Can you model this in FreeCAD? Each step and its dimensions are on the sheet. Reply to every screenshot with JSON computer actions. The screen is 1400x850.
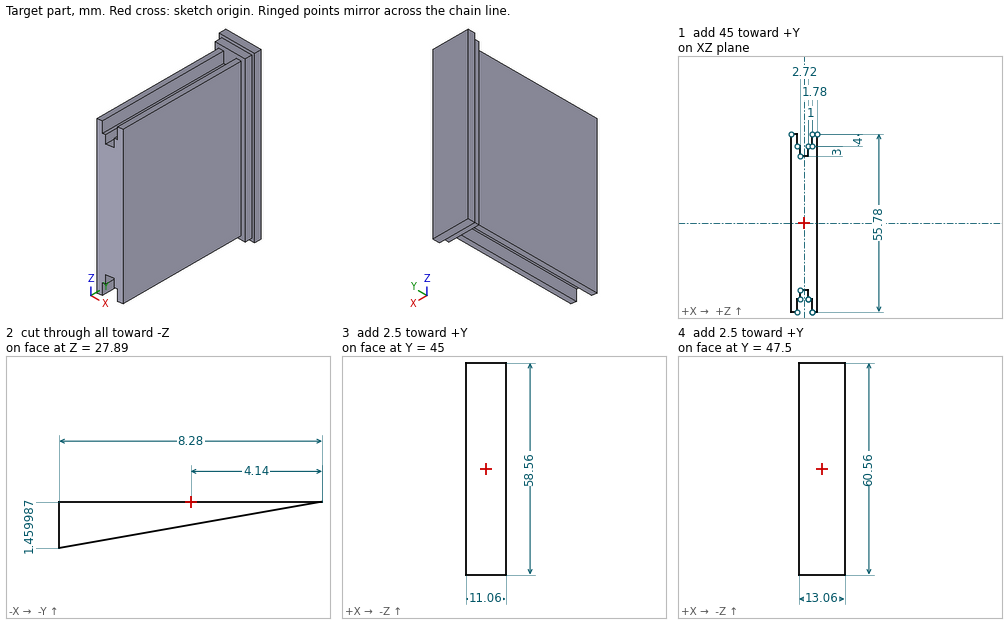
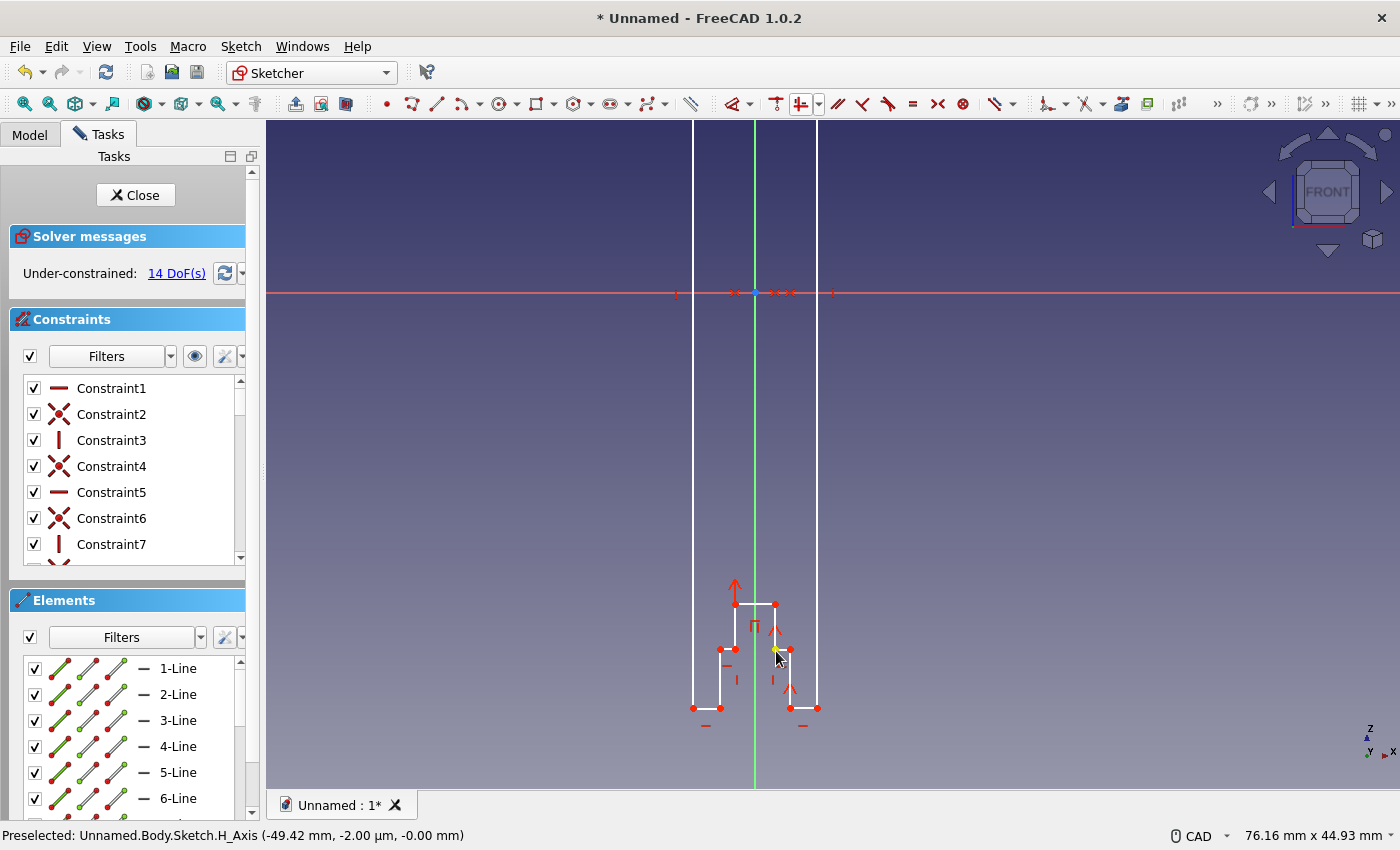
{"action": "left_click", "coordinate": [775, 650]}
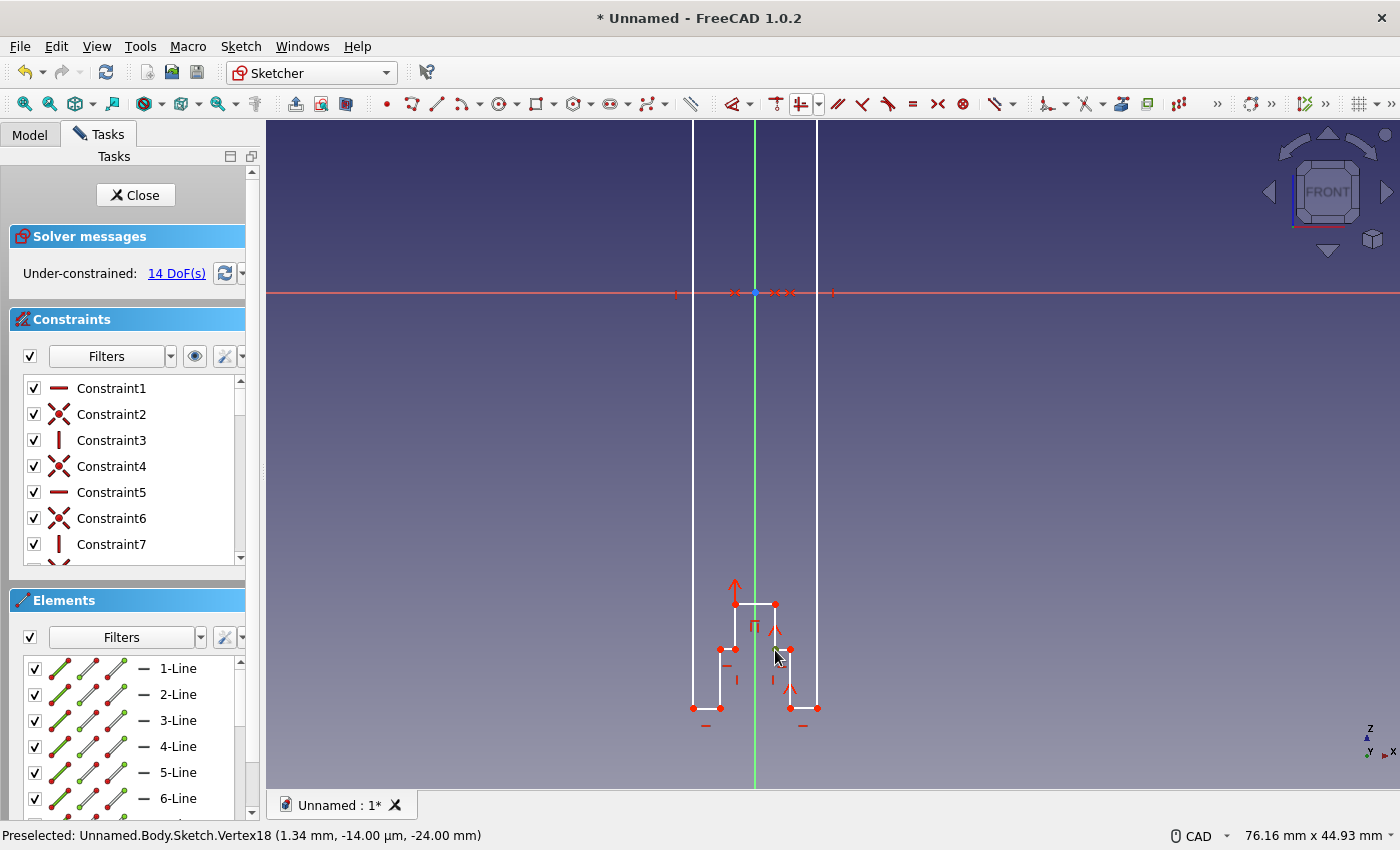
{"action": "left_click", "coordinate": [735, 649]}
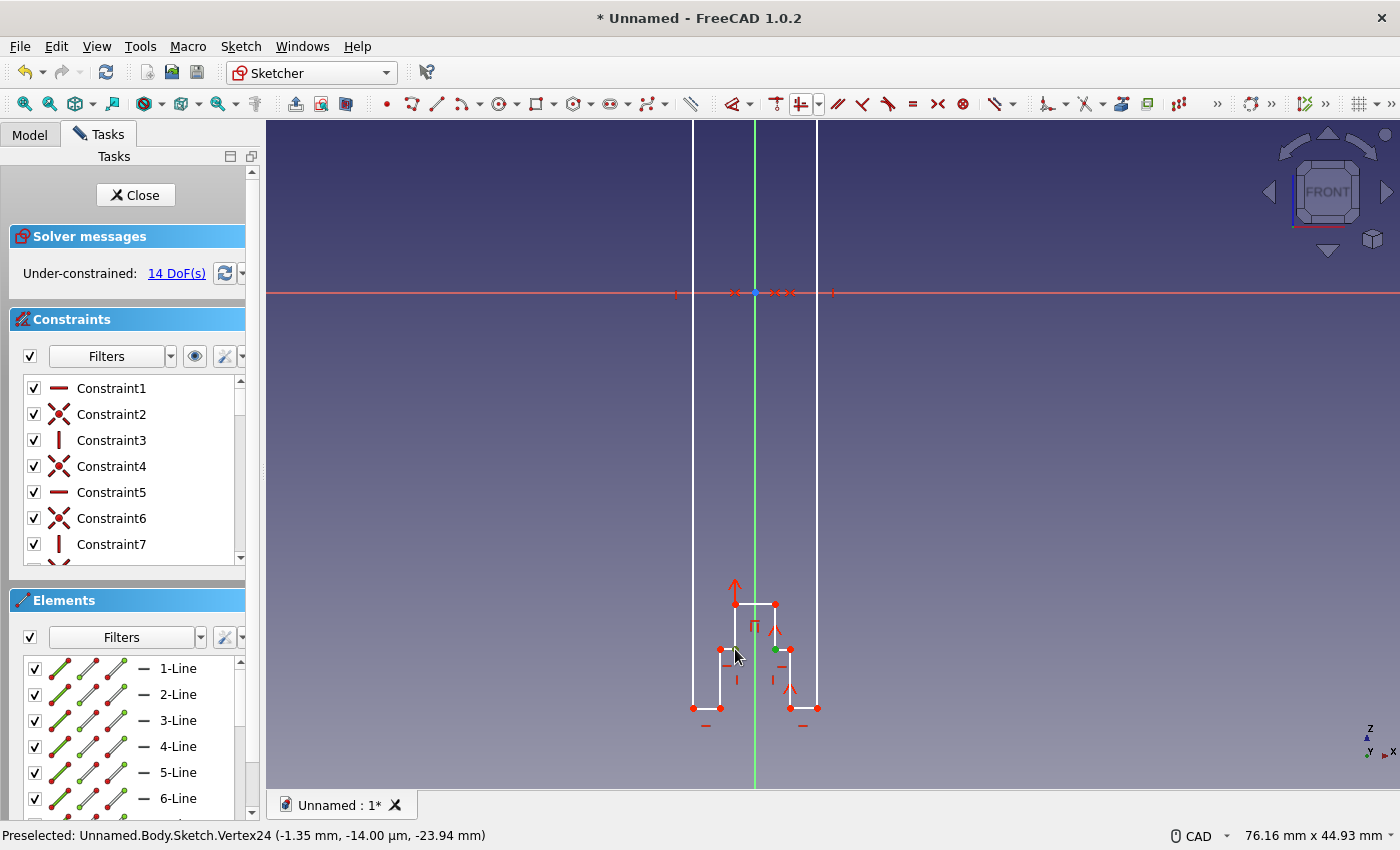
{"action": "left_click", "coordinate": [755, 717]}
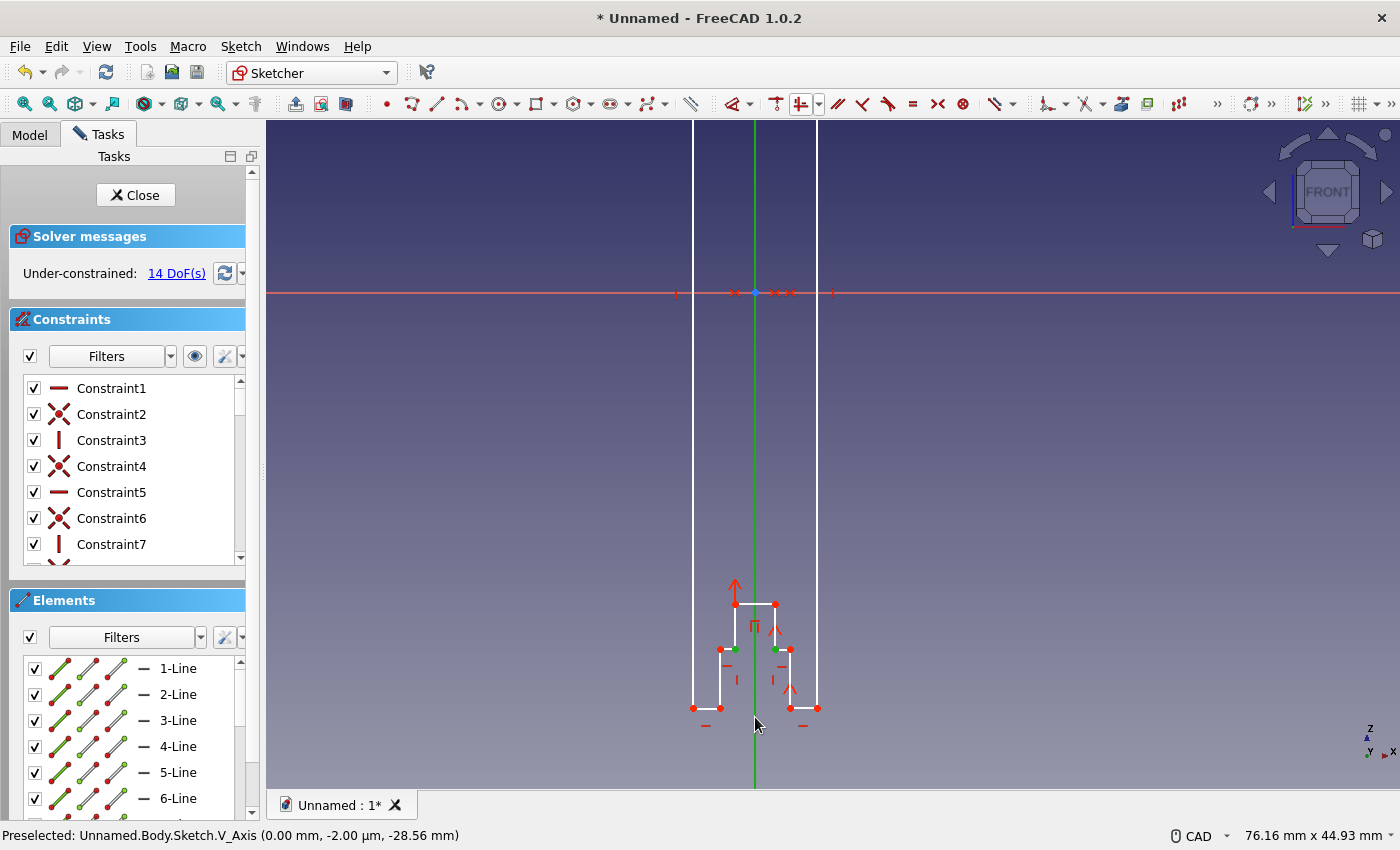
{"action": "left_click", "coordinate": [938, 104]}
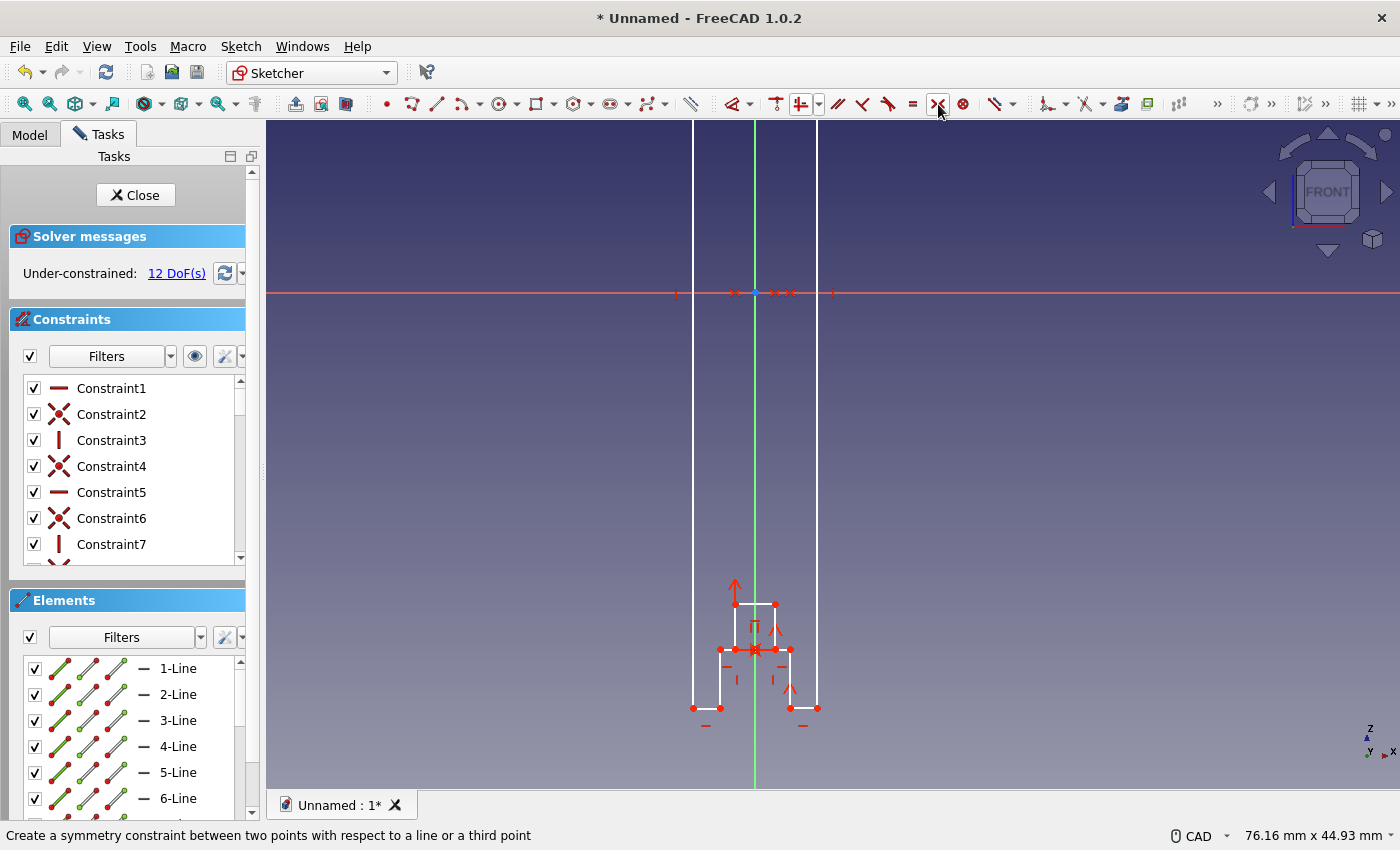
{"action": "left_click", "coordinate": [790, 708]}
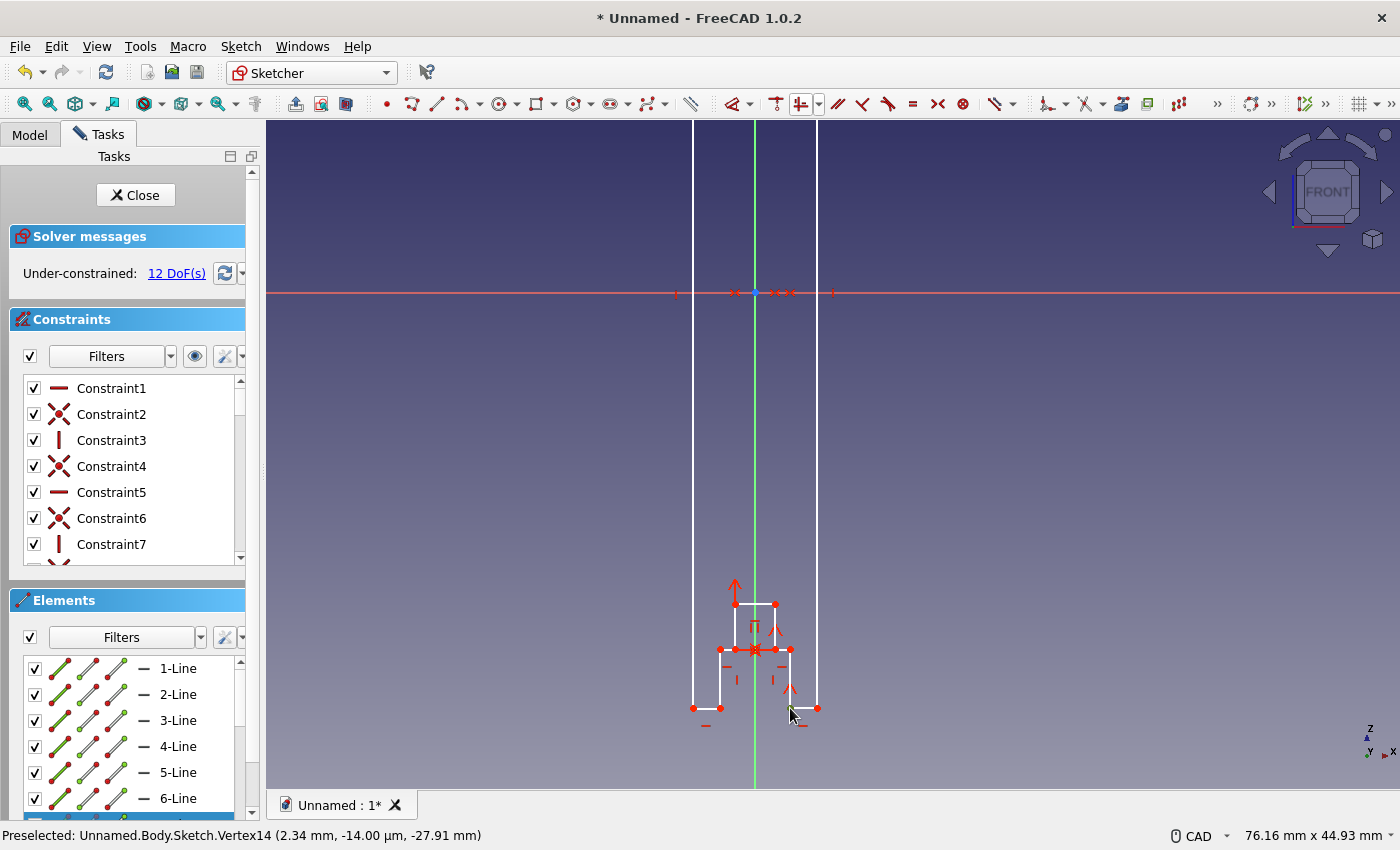
{"action": "left_click", "coordinate": [720, 709]}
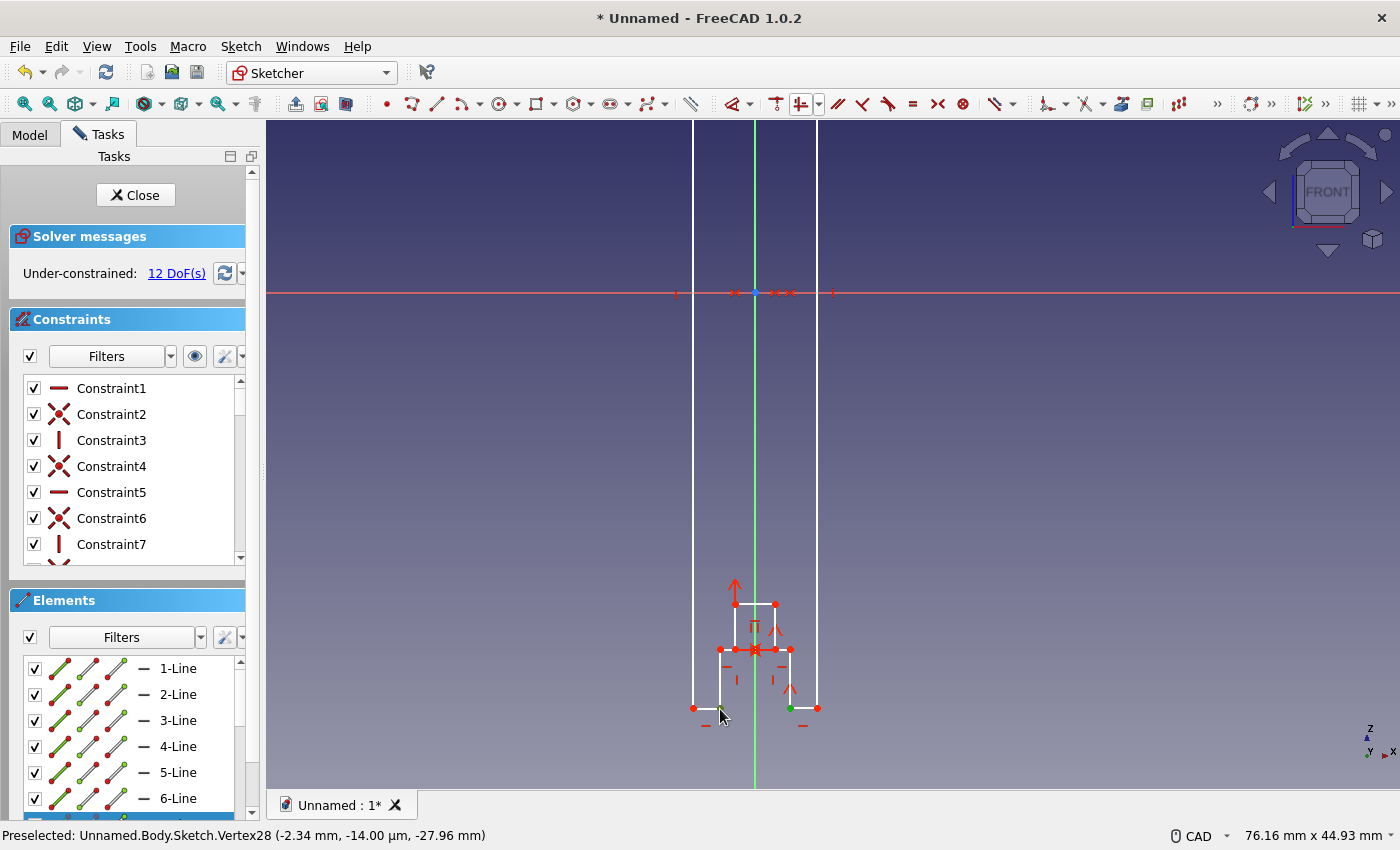
{"action": "left_click", "coordinate": [755, 717]}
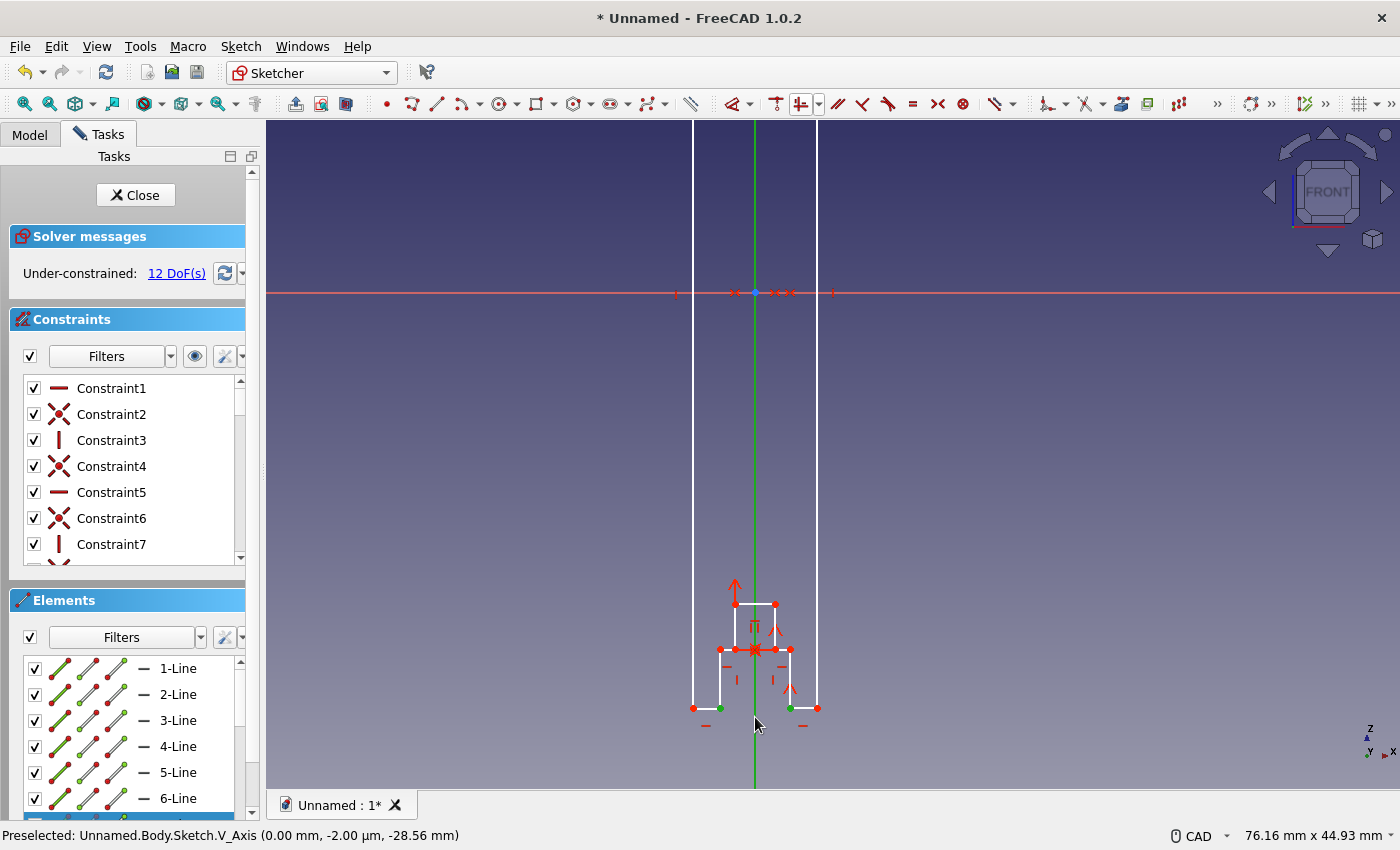
{"action": "key", "text": "s"}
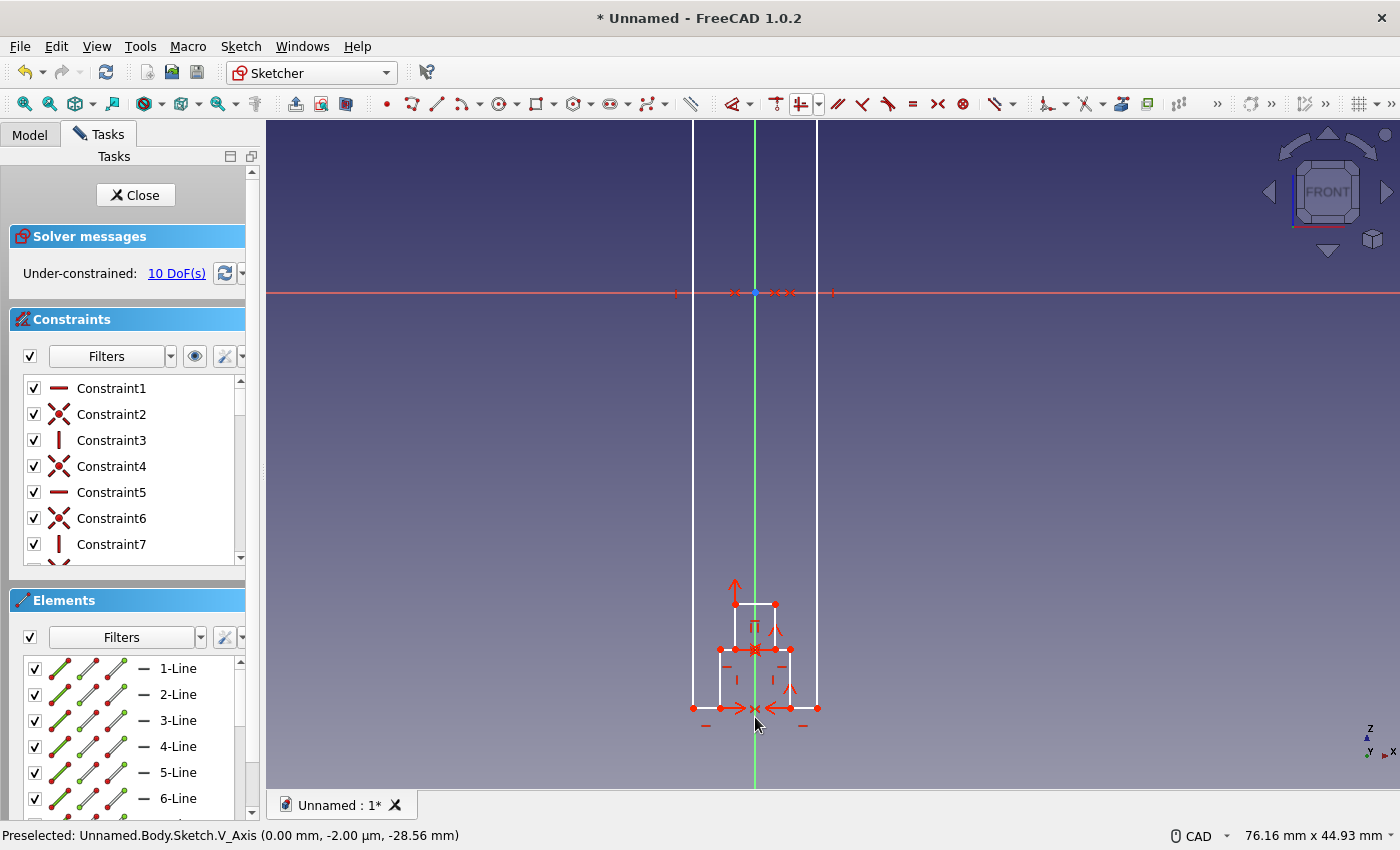
{"action": "scroll", "coordinate": [776, 651], "scroll_direction": "down", "scroll_amount": 3}